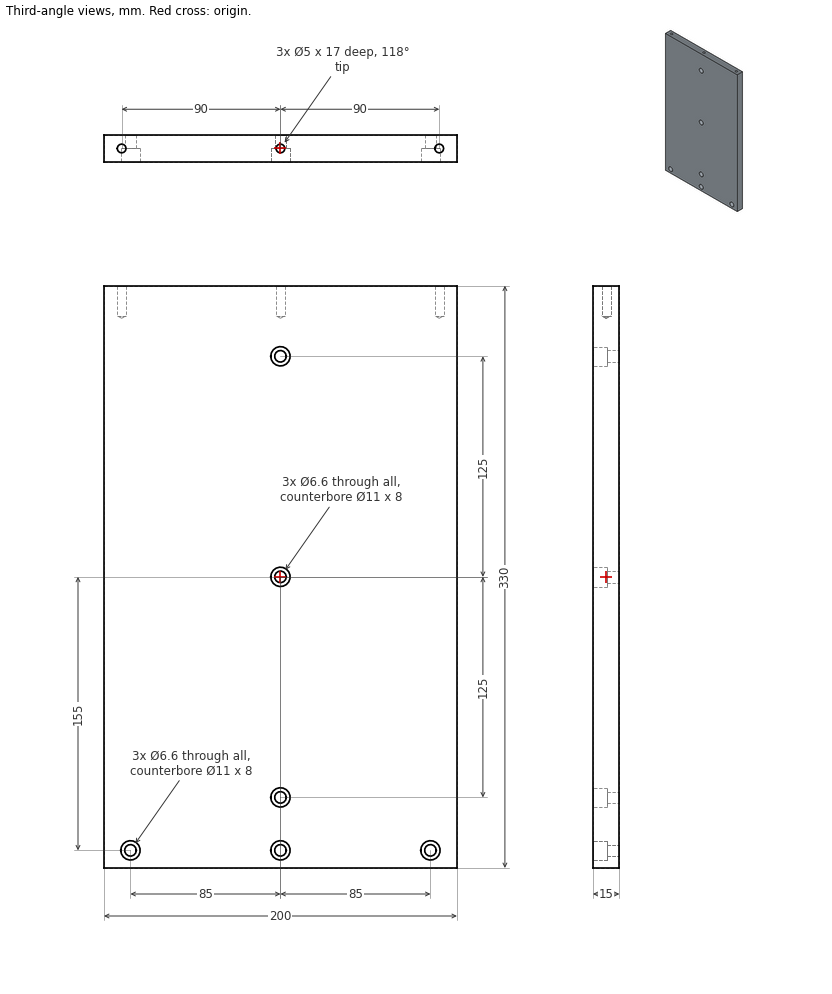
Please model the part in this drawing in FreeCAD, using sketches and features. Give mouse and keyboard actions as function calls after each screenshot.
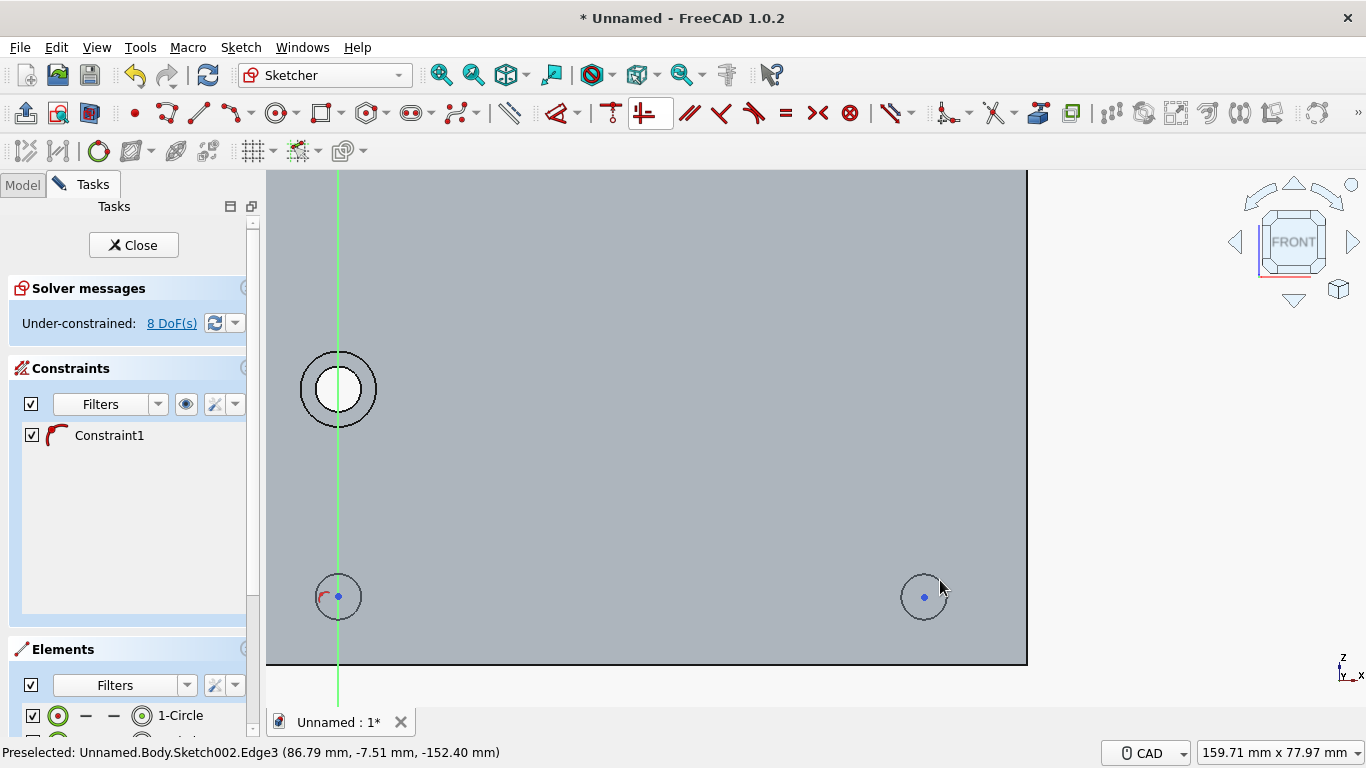
scroll(924, 596, down, 6)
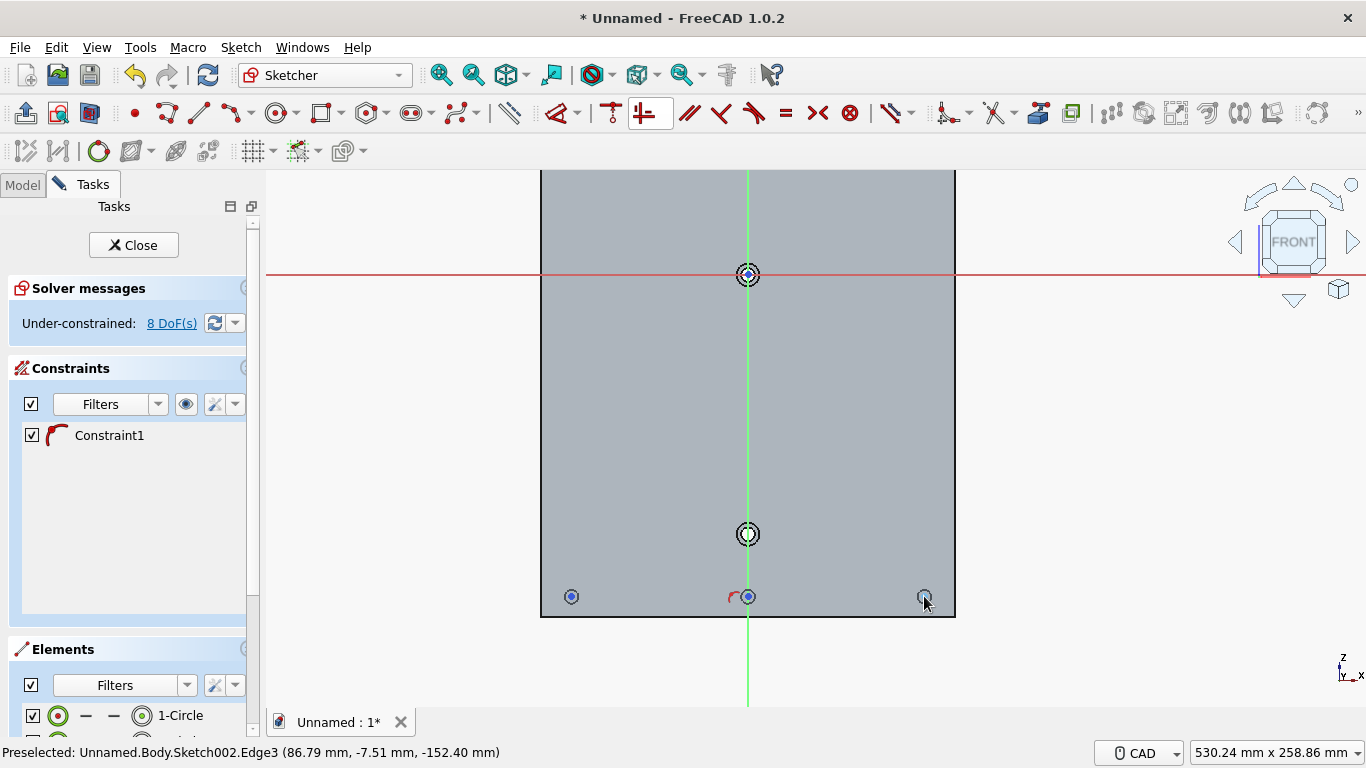
scroll(576, 592, up, 4)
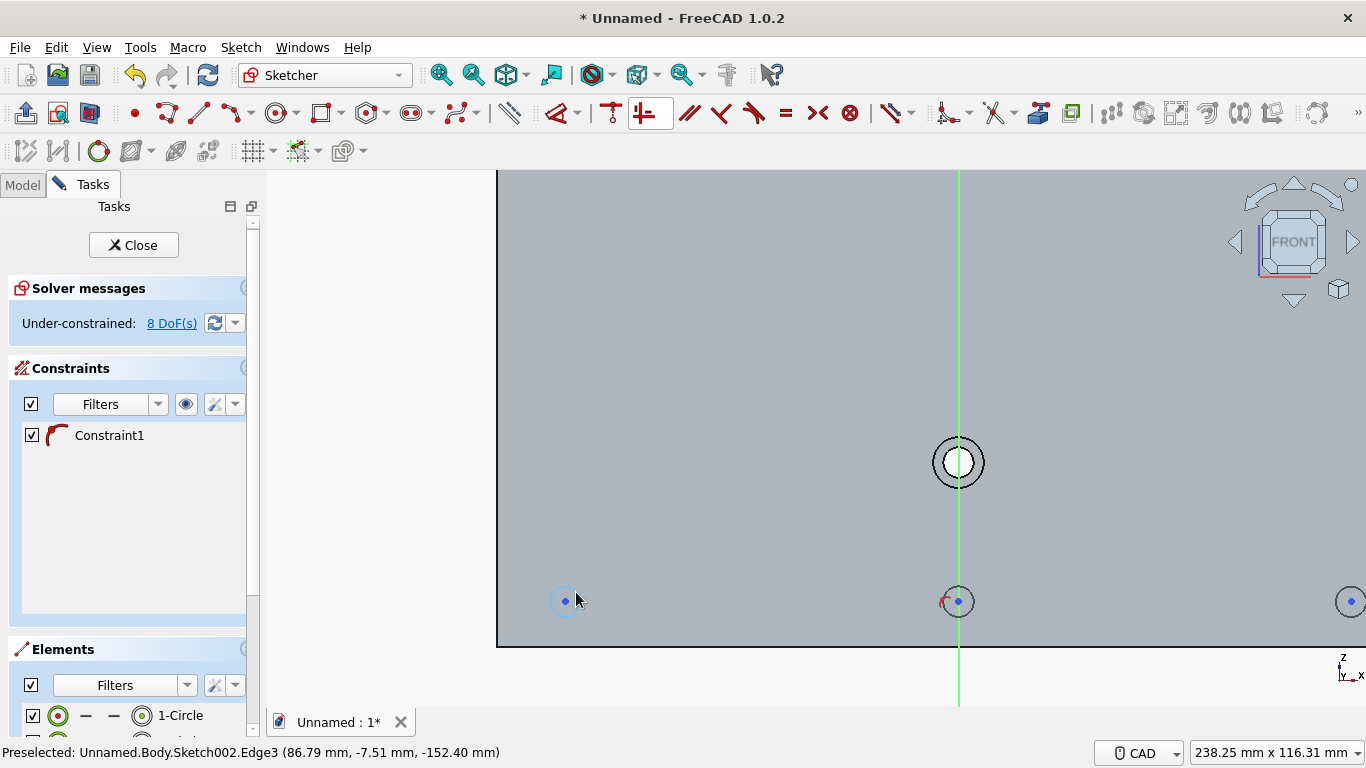
click(577, 591)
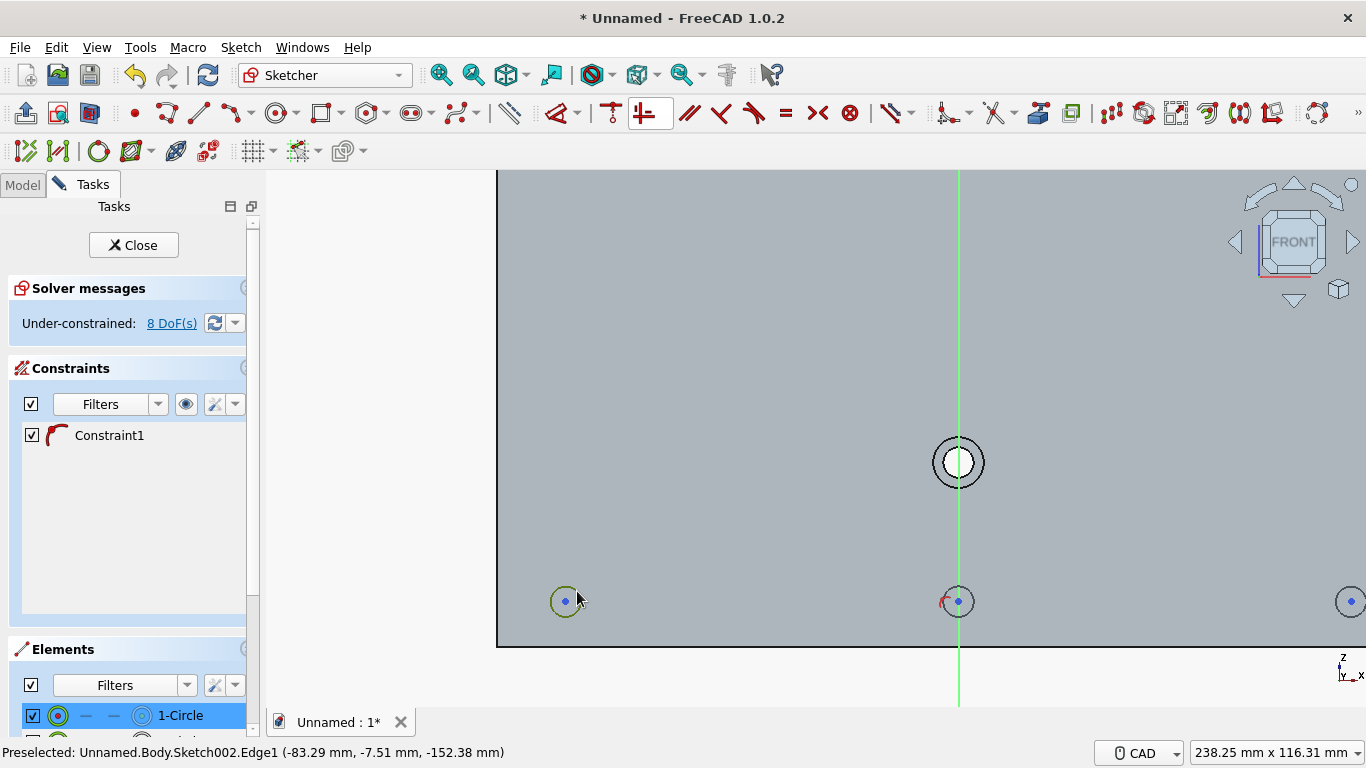
scroll(969, 591, up, 2)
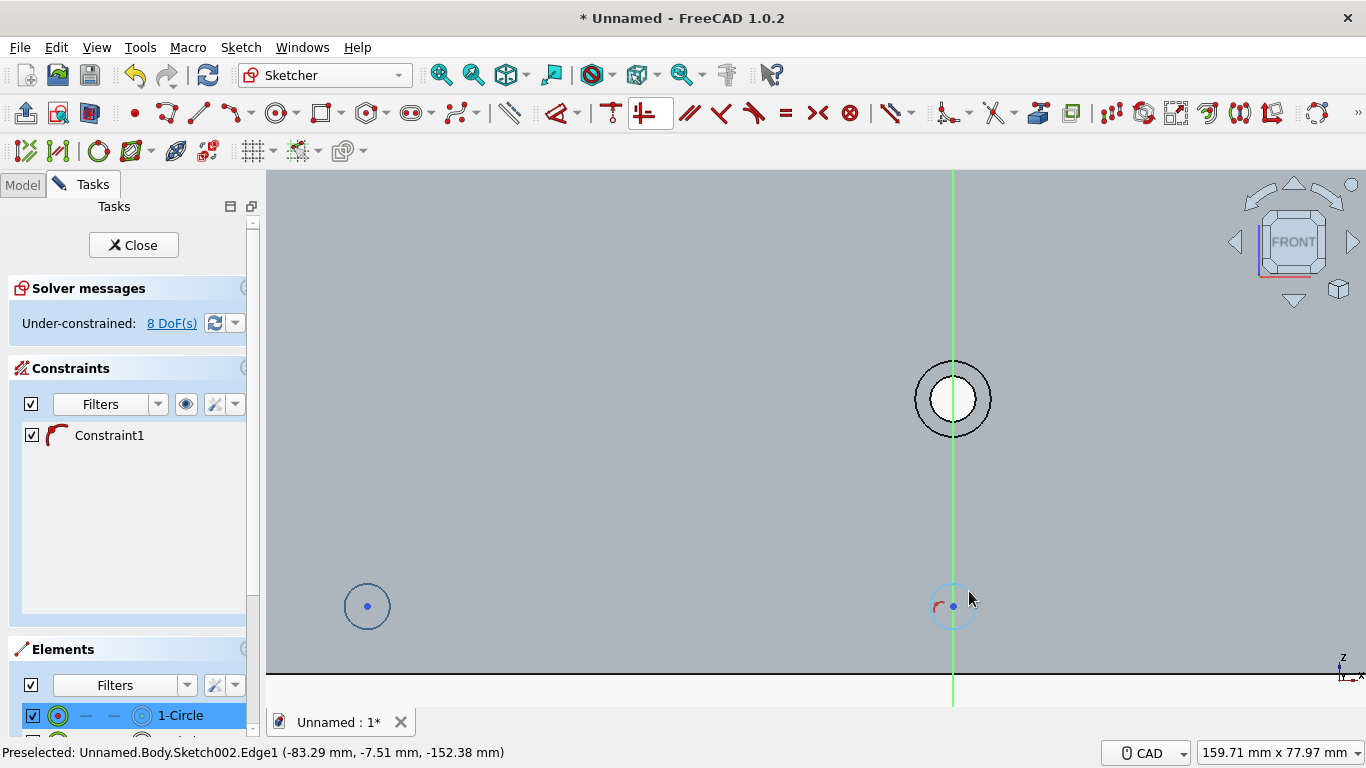
click(969, 590)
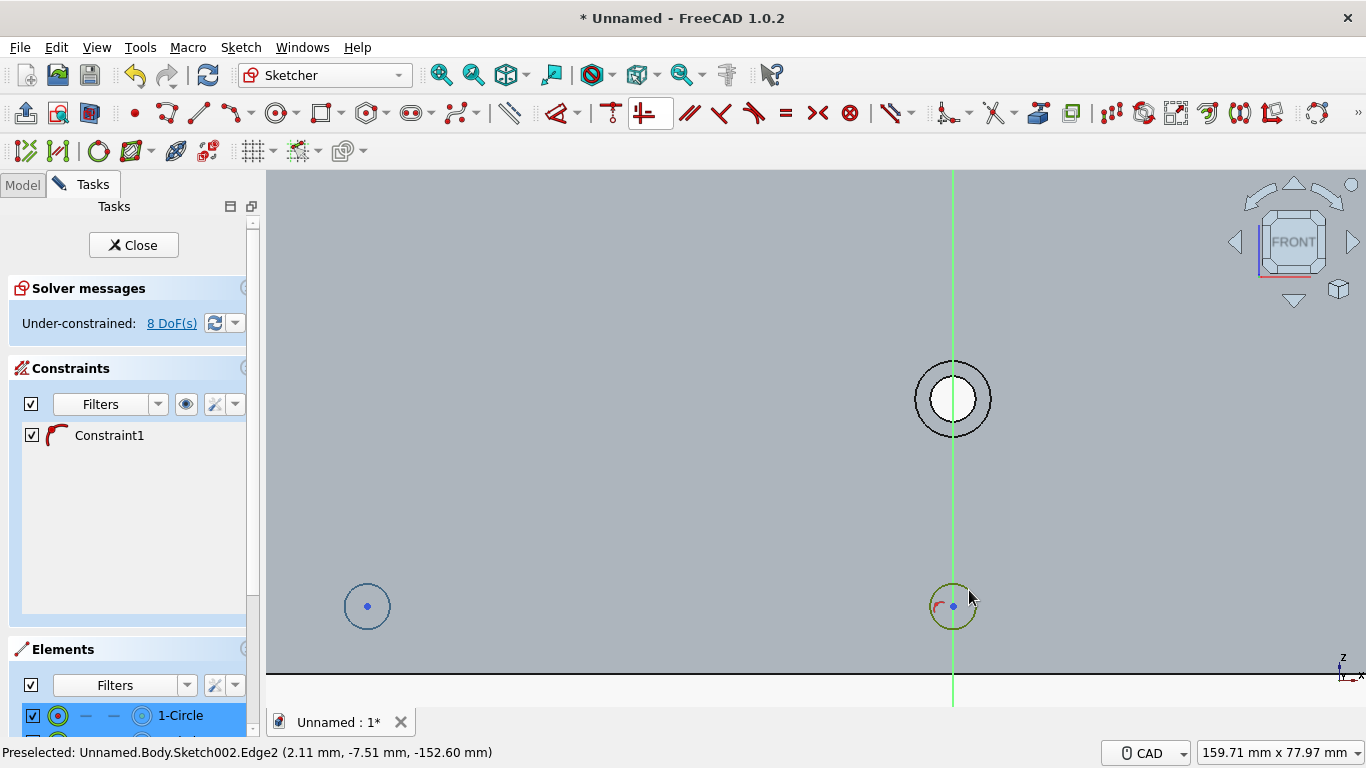
scroll(659, 592, down, 6)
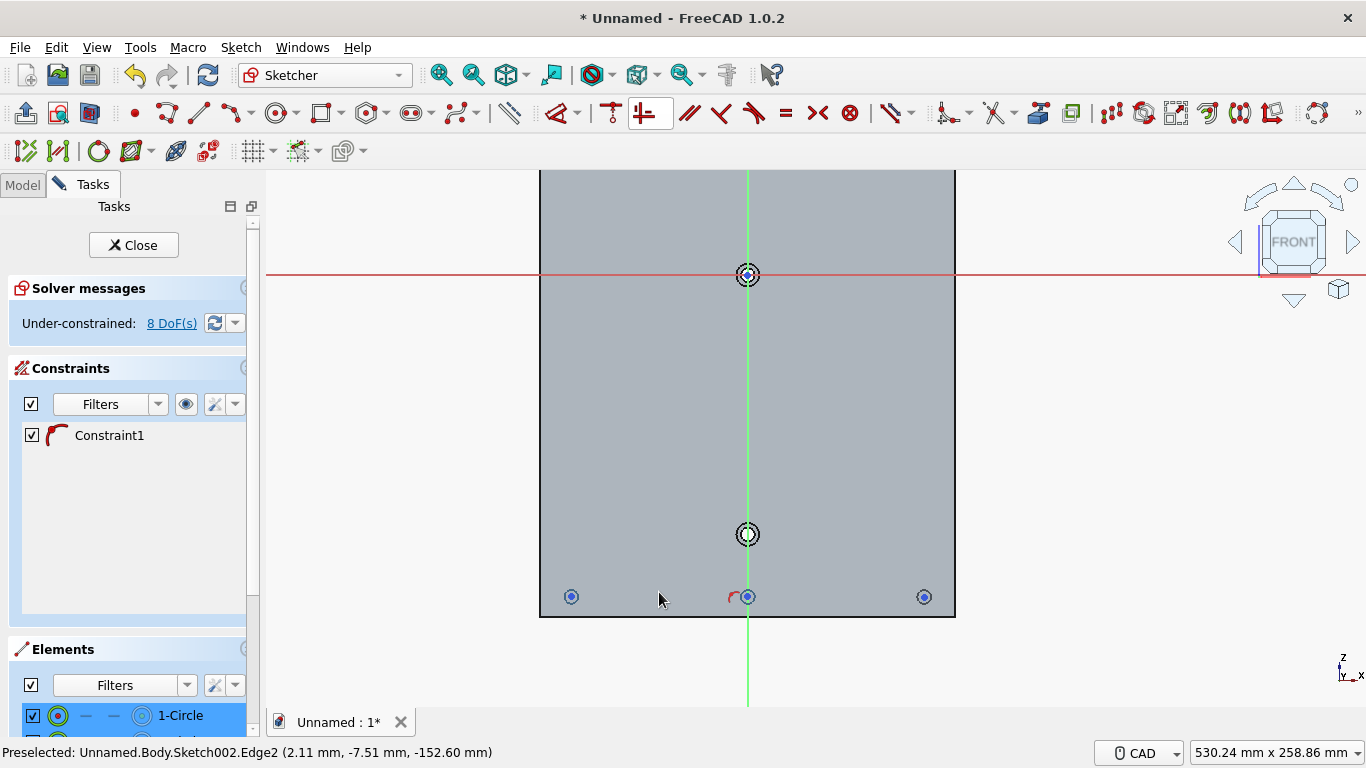
scroll(929, 592, up, 4)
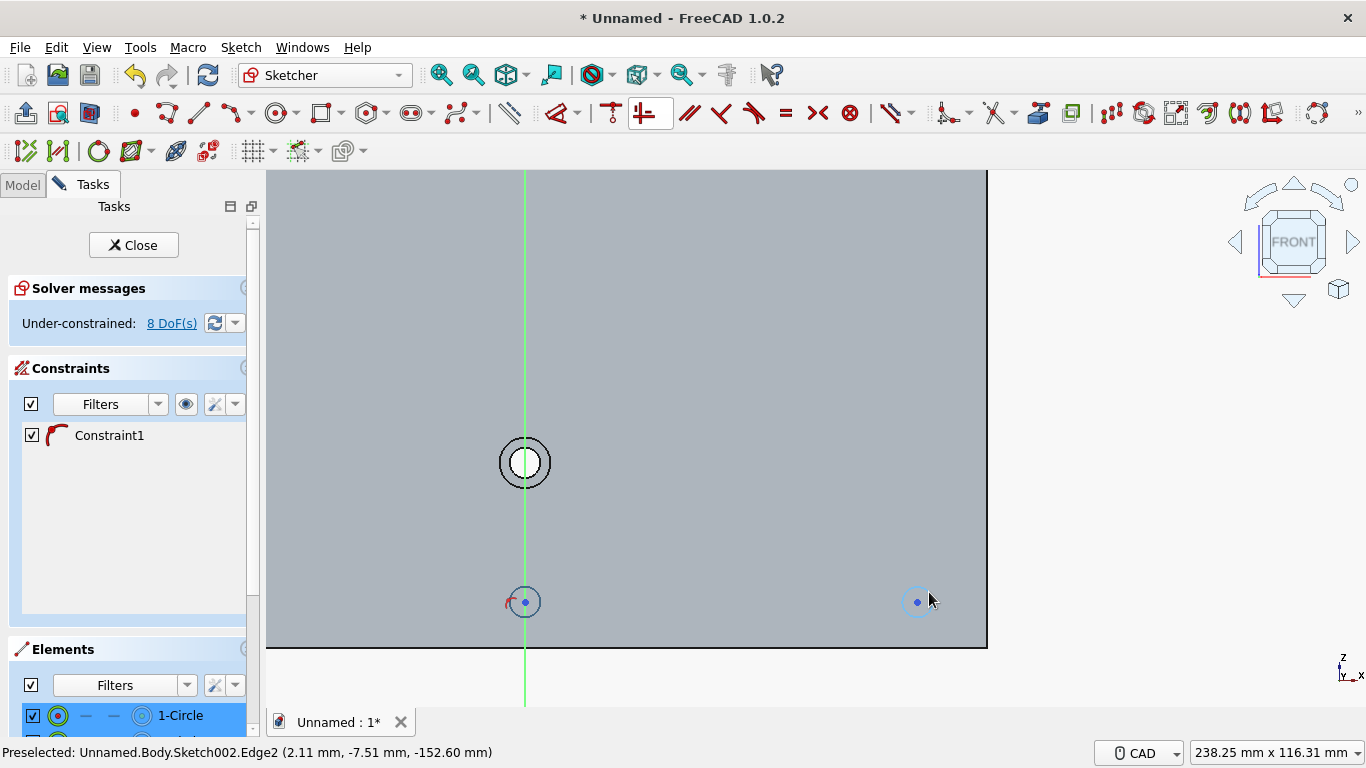
click(928, 591)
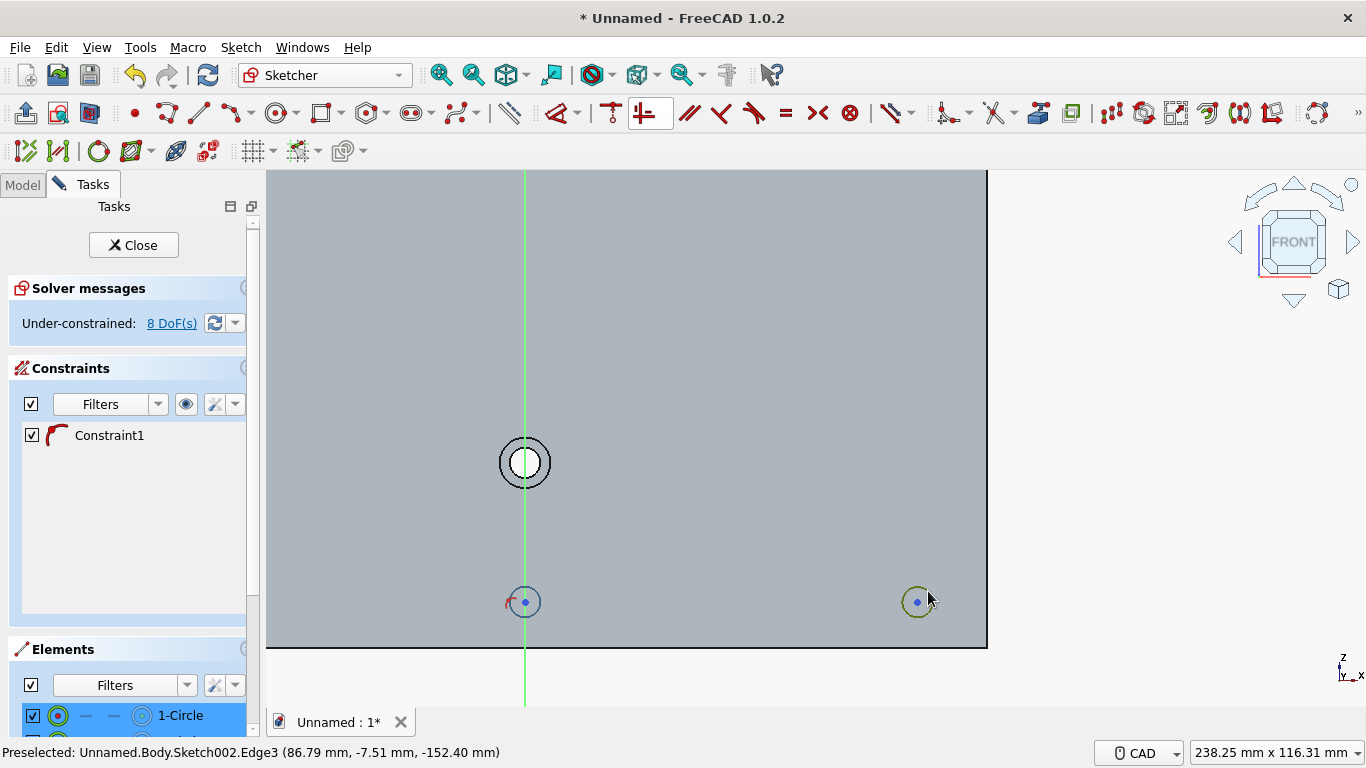
click(786, 114)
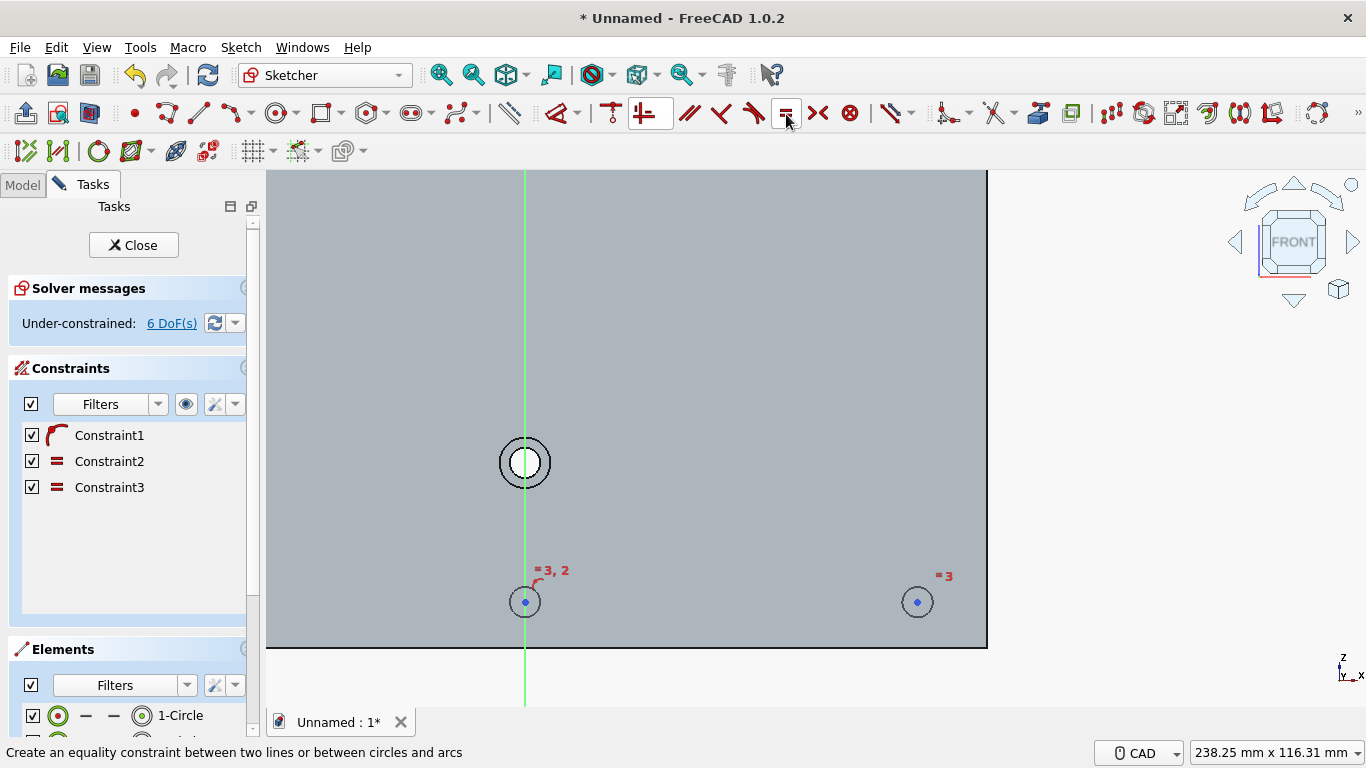
scroll(929, 591, down, 4)